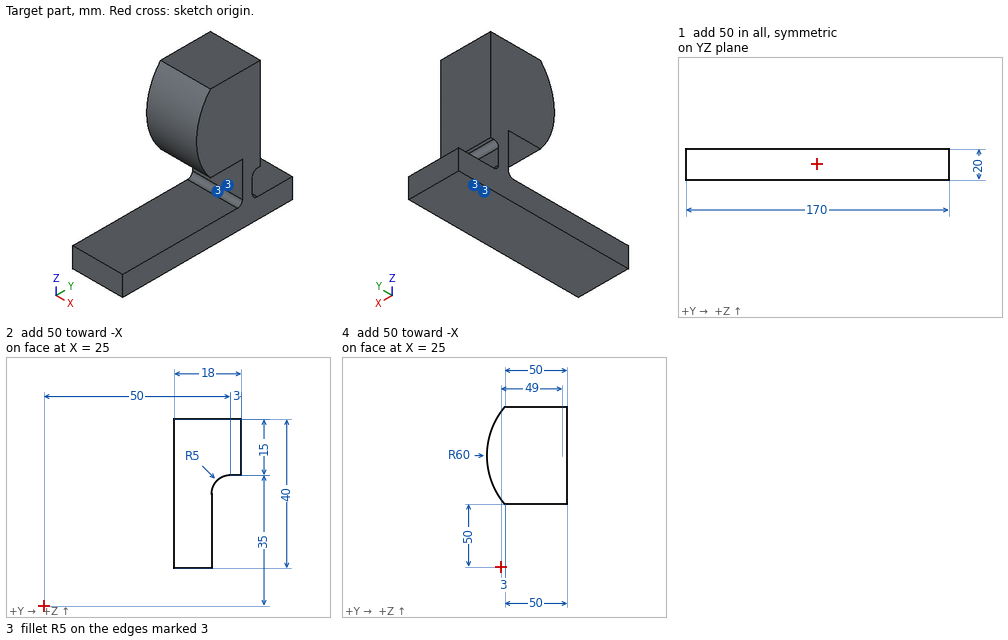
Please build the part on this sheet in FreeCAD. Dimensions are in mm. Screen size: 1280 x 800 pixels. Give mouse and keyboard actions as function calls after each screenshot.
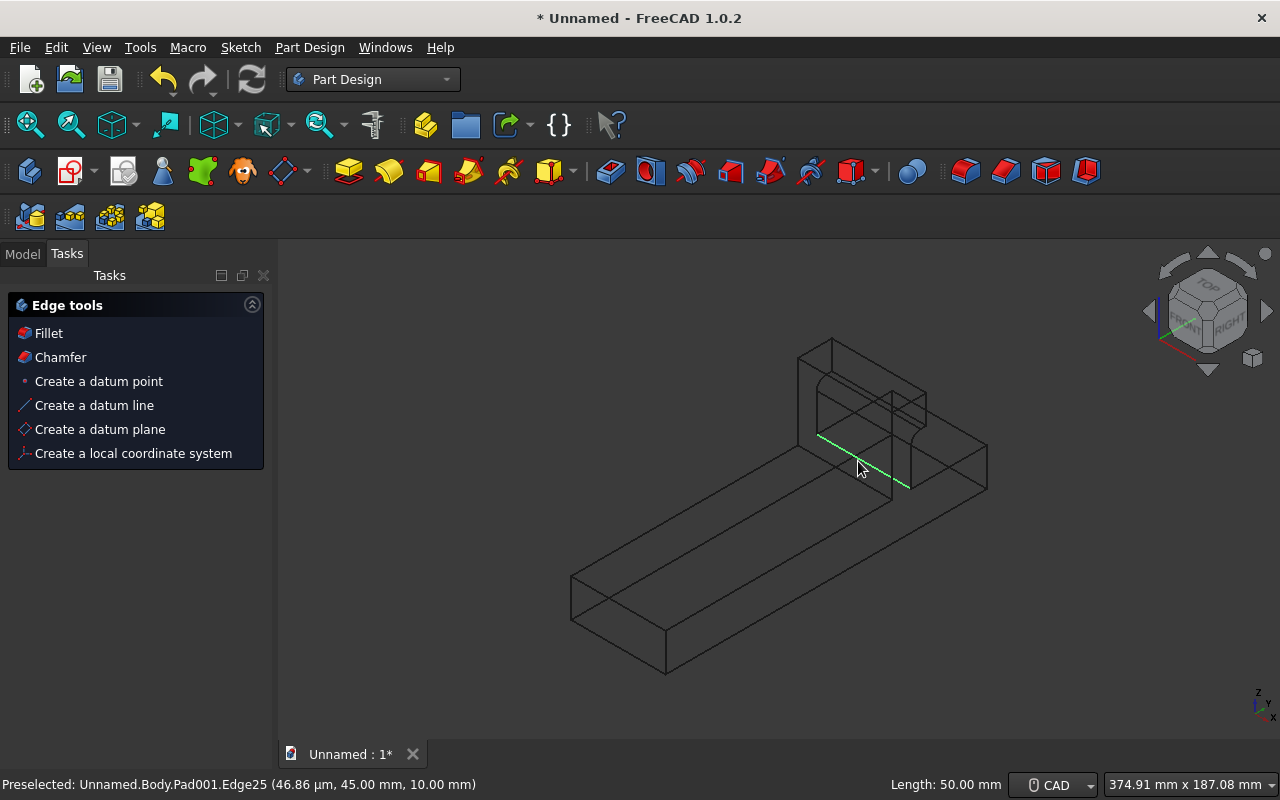
click(845, 472, ctrl)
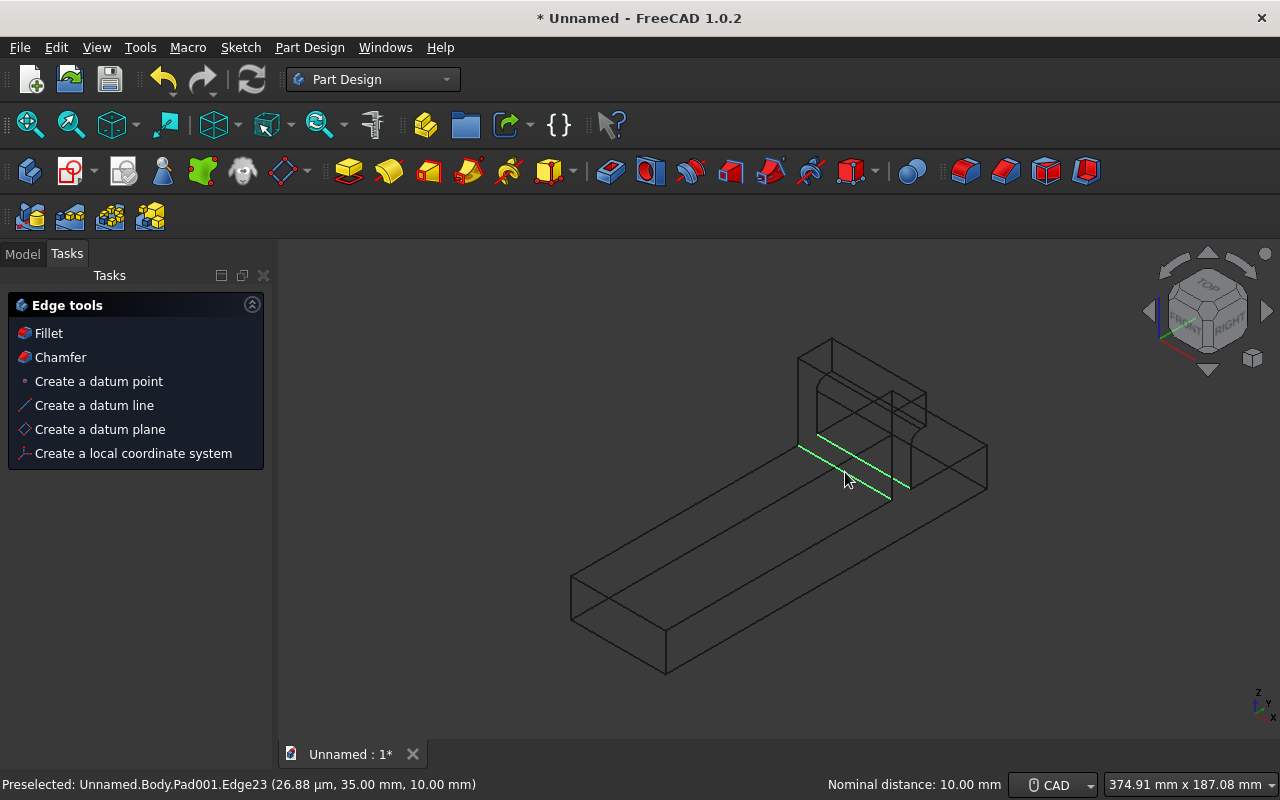
key(v)
key(1)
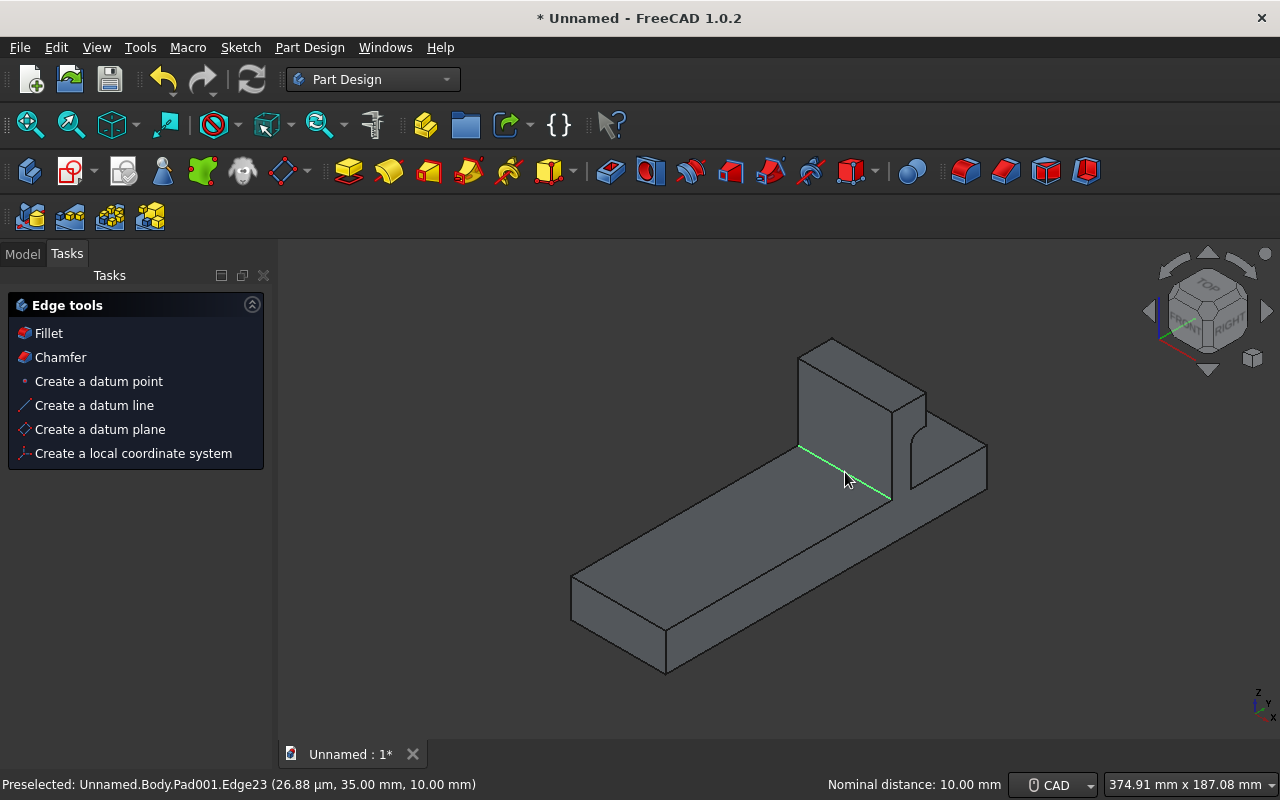
click(966, 172)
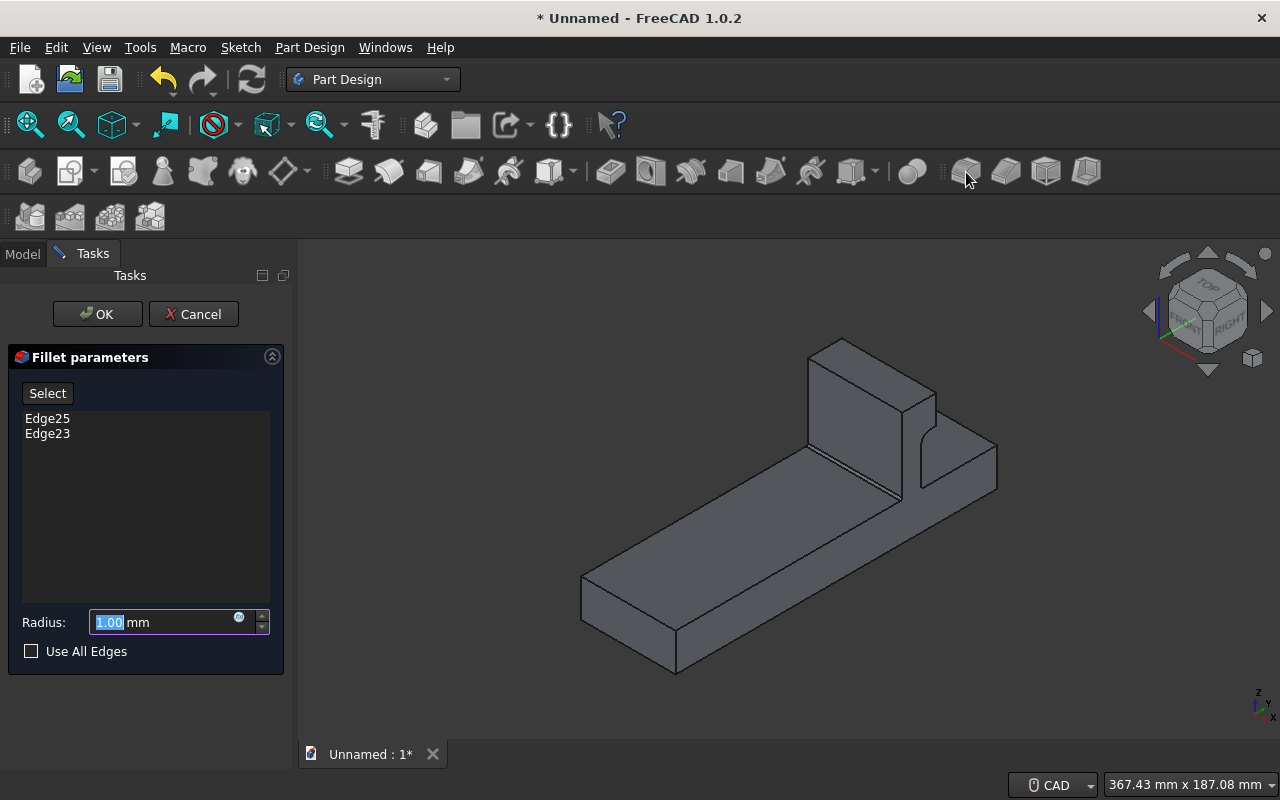
text(5)
key(Tab)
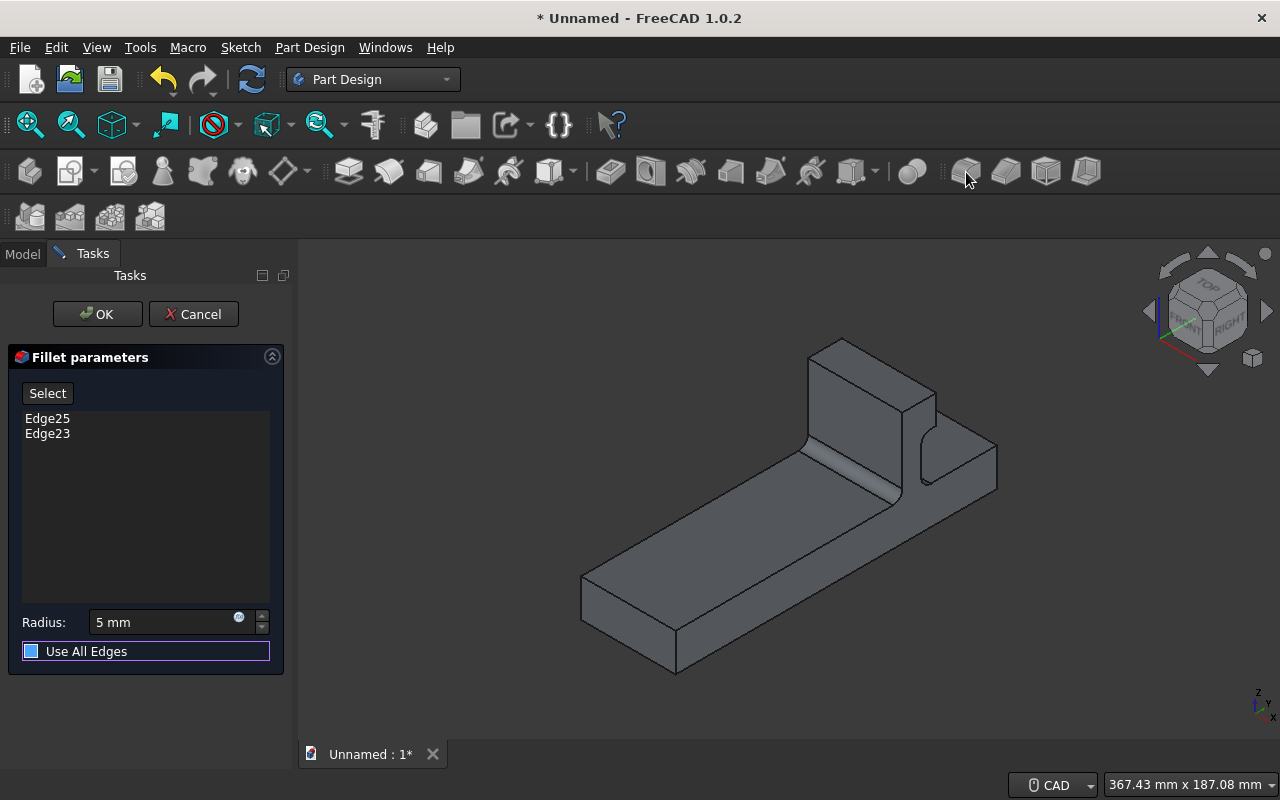
click(98, 314)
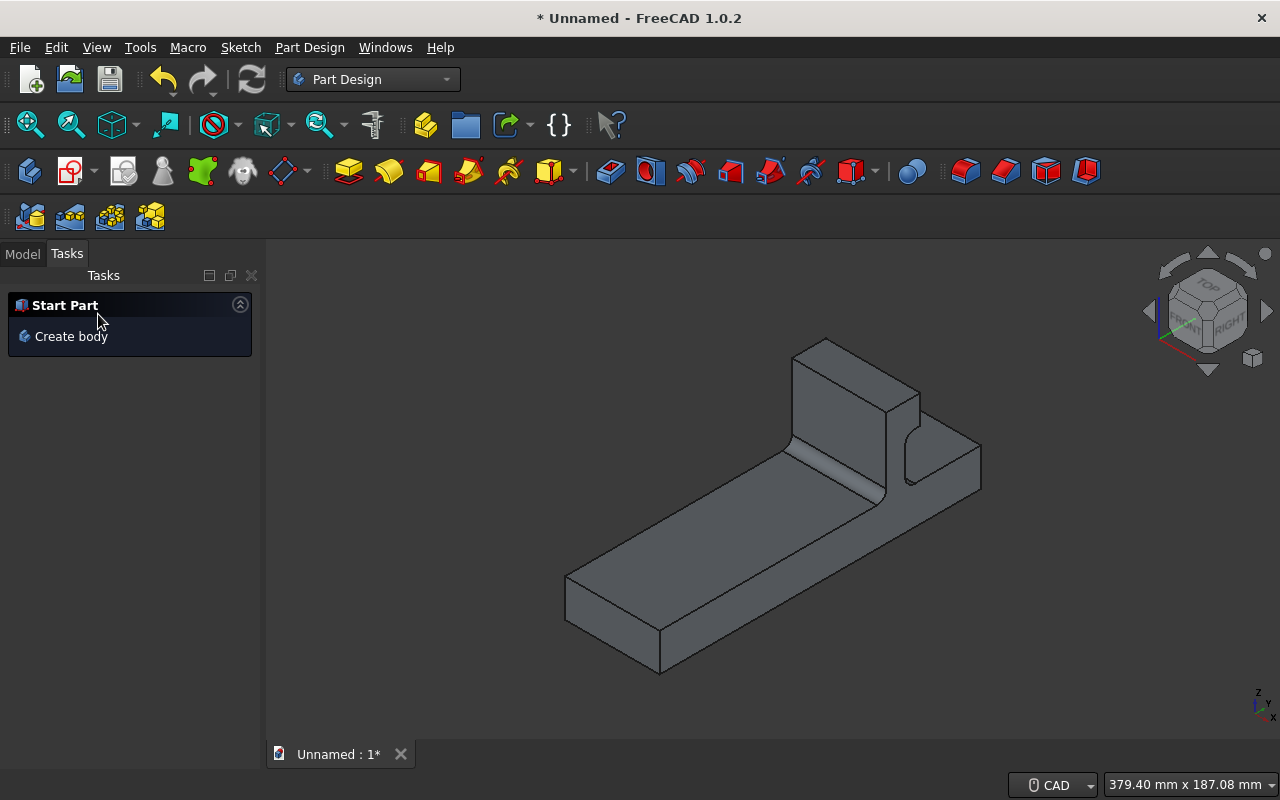
click(912, 500)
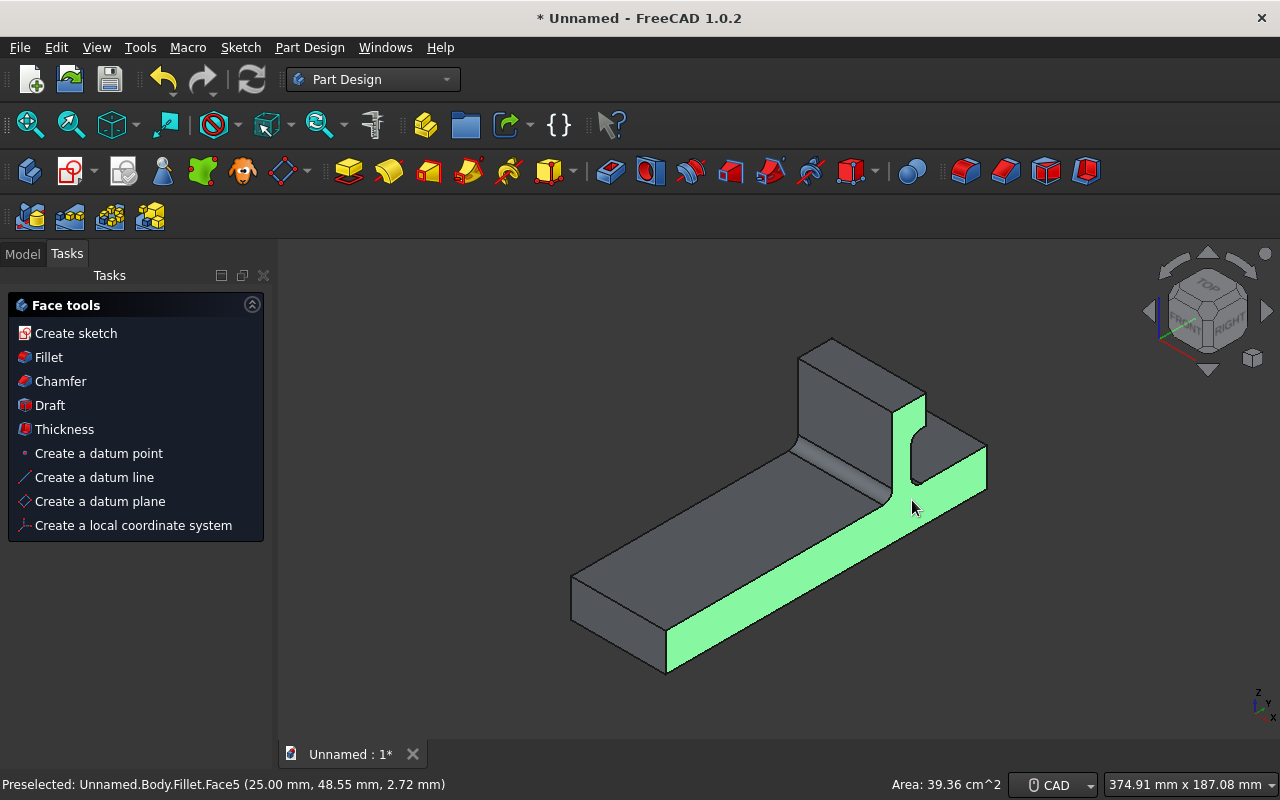
click(70, 172)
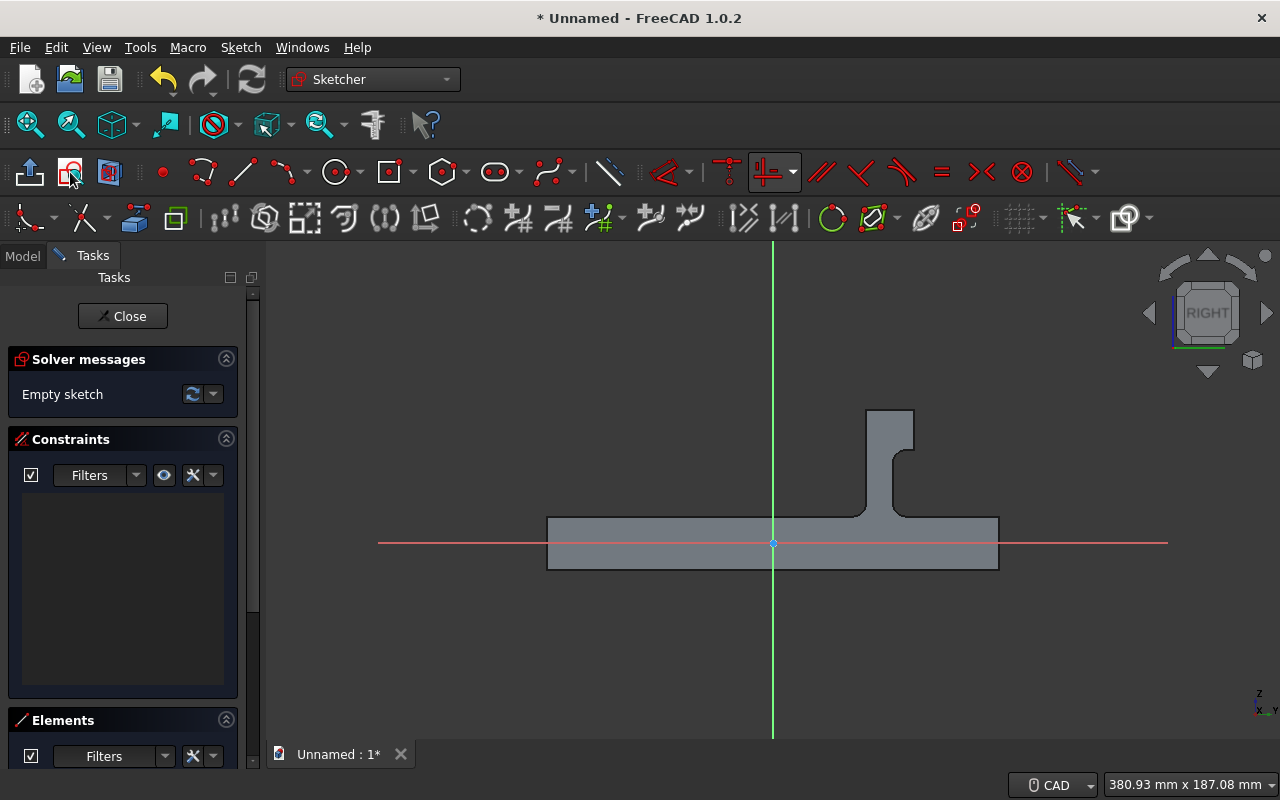
scroll(294, 711, down, 1)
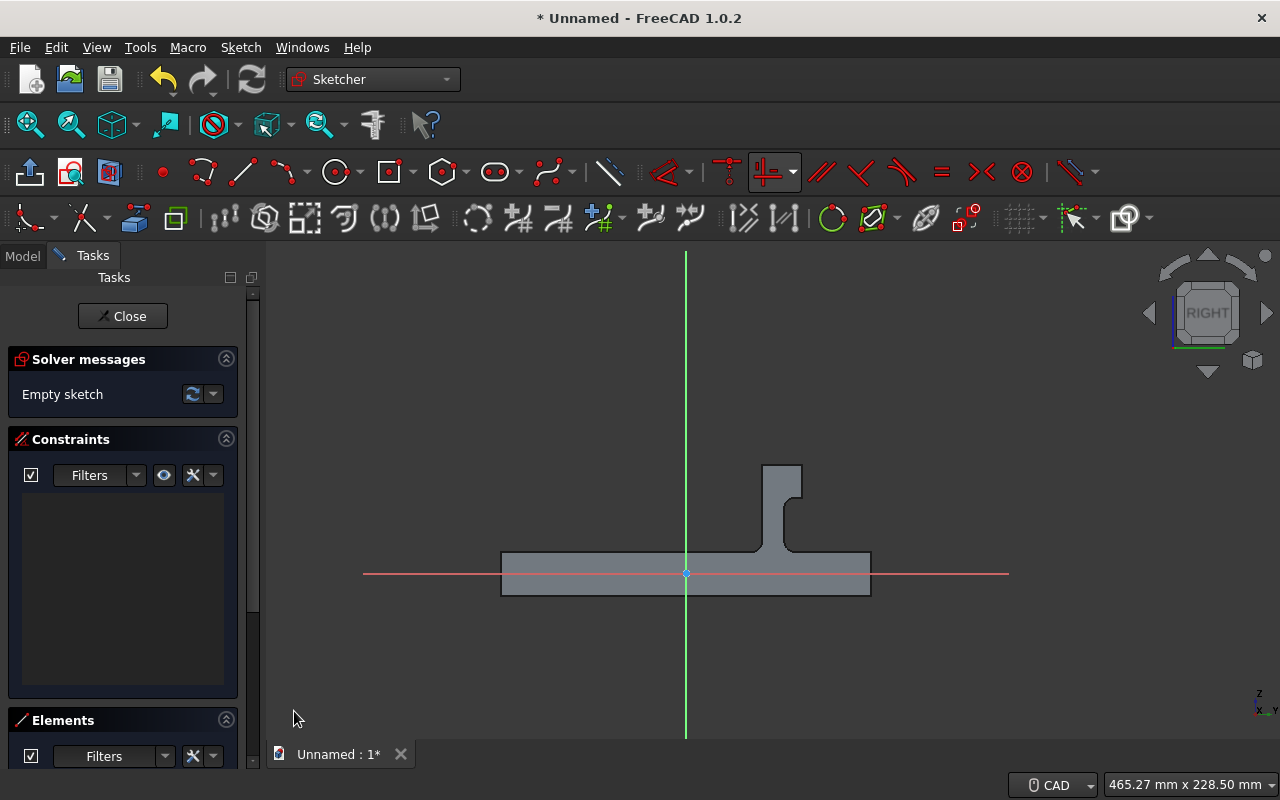
key(g)
key(m)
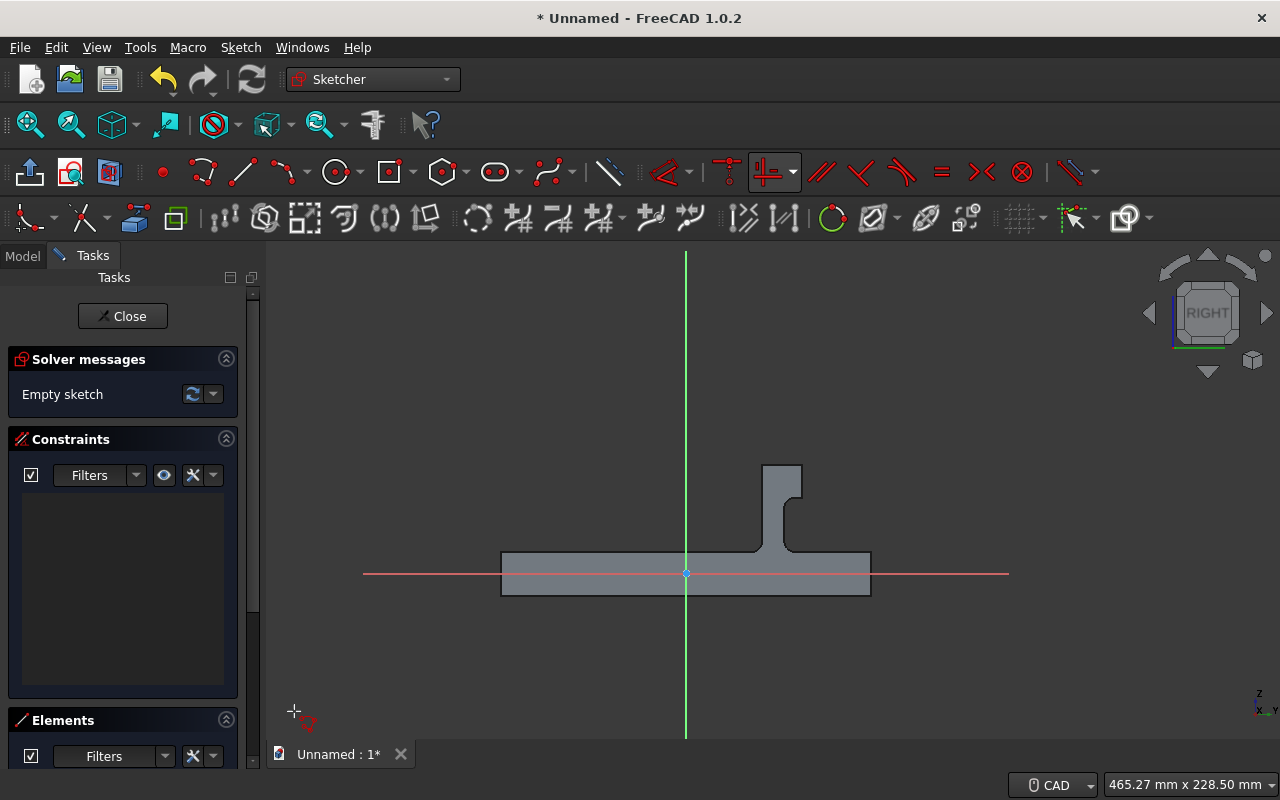
scroll(693, 465, up, 5)